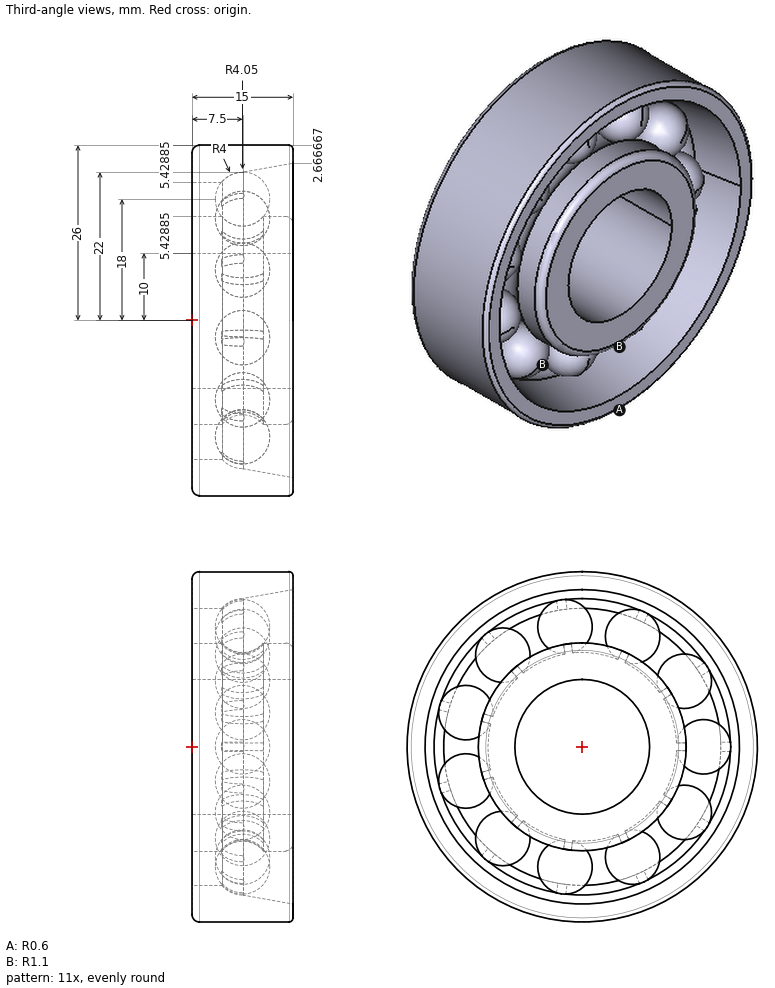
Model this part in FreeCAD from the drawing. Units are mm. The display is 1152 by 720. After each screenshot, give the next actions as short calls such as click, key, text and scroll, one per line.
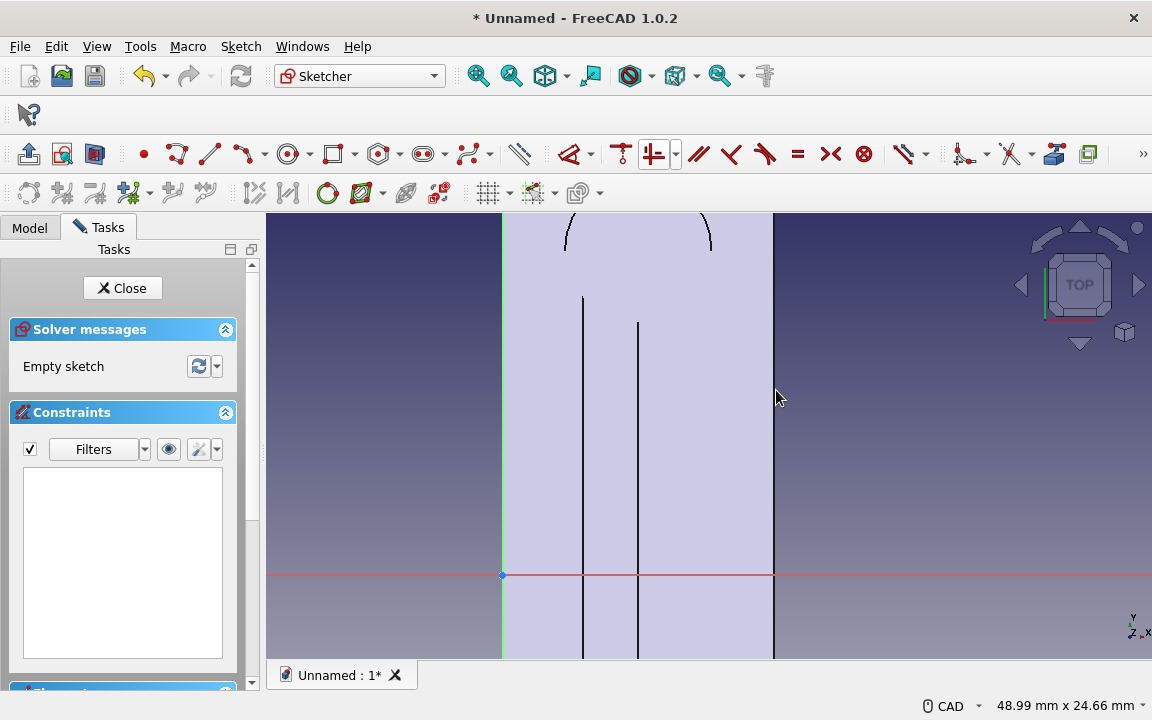
key(g)
key(m)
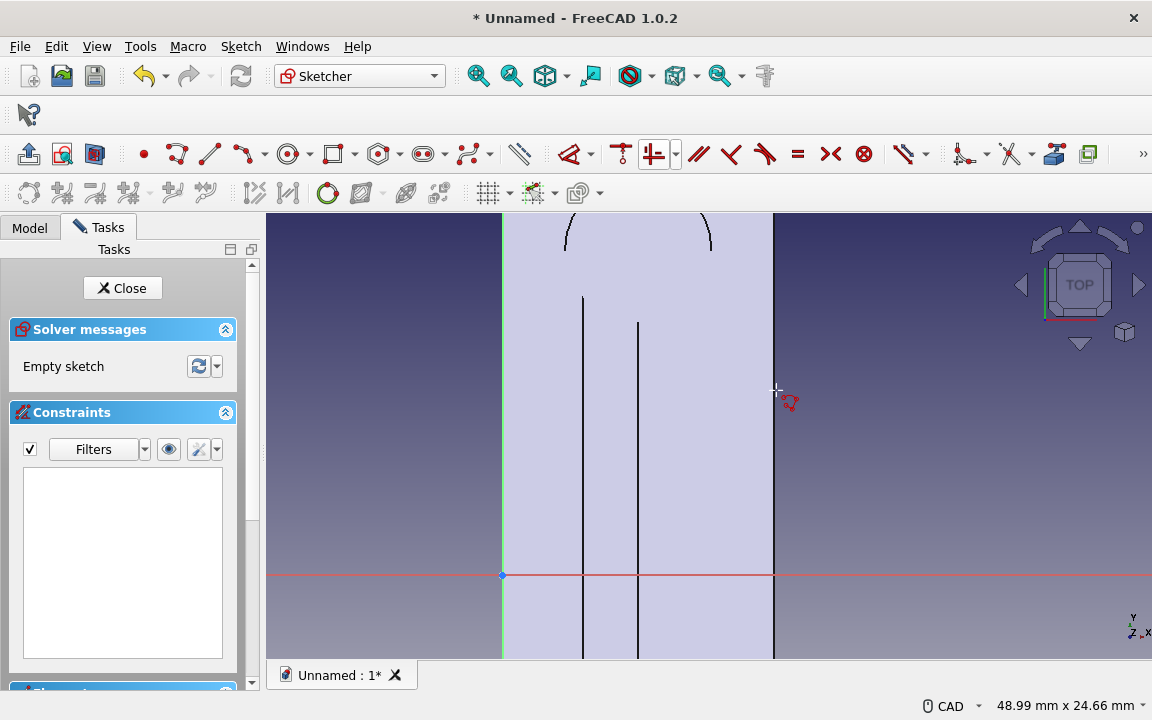
click(583, 296)
click(503, 296)
click(512, 394)
click(774, 394)
click(774, 296)
click(694, 296)
right_click(694, 296)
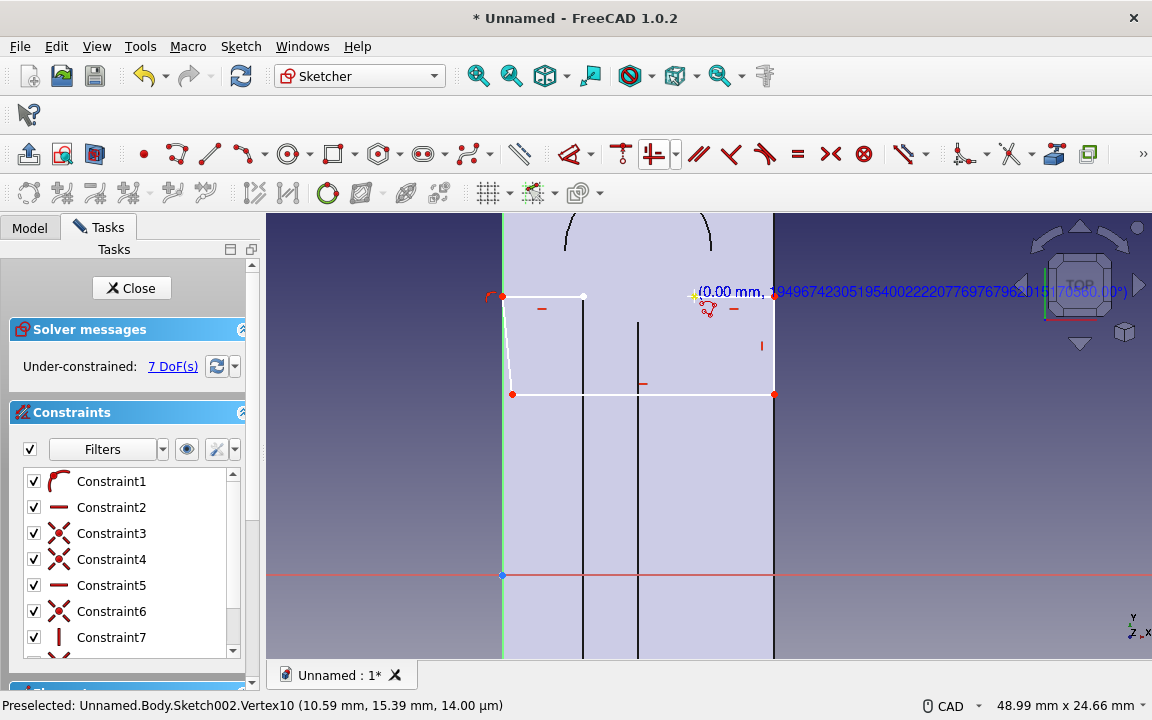
click(242, 154)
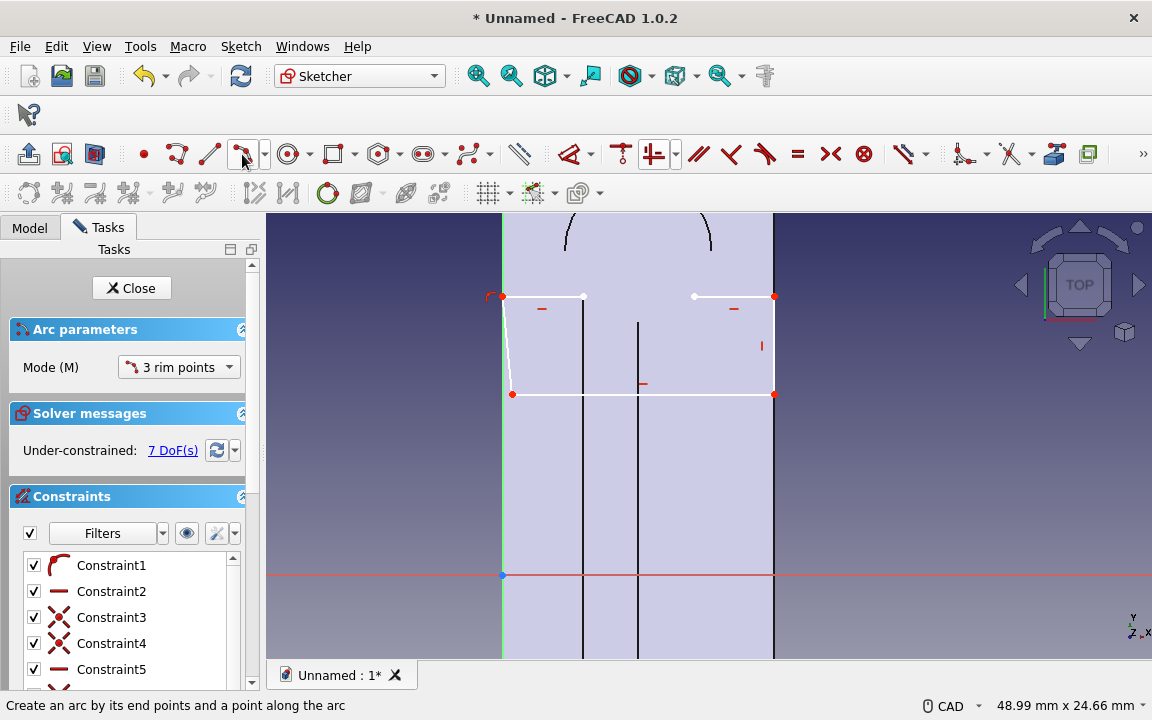
click(694, 297)
click(583, 297)
click(638, 322)
key(Escape)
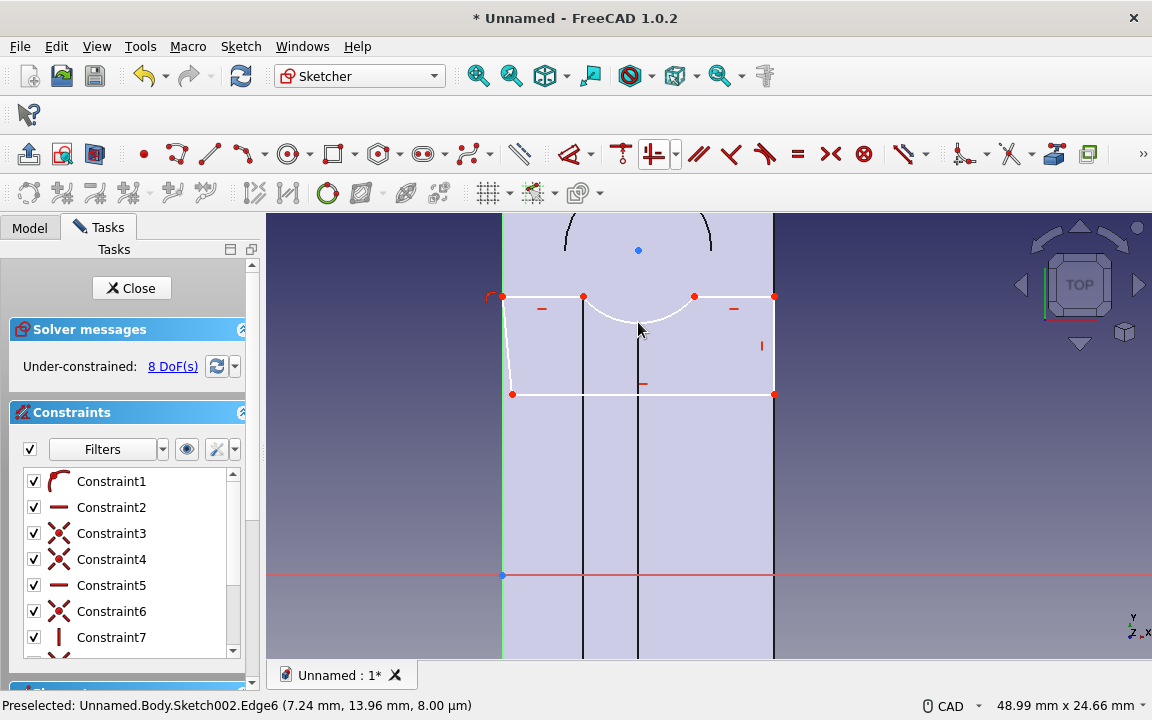
click(505, 326)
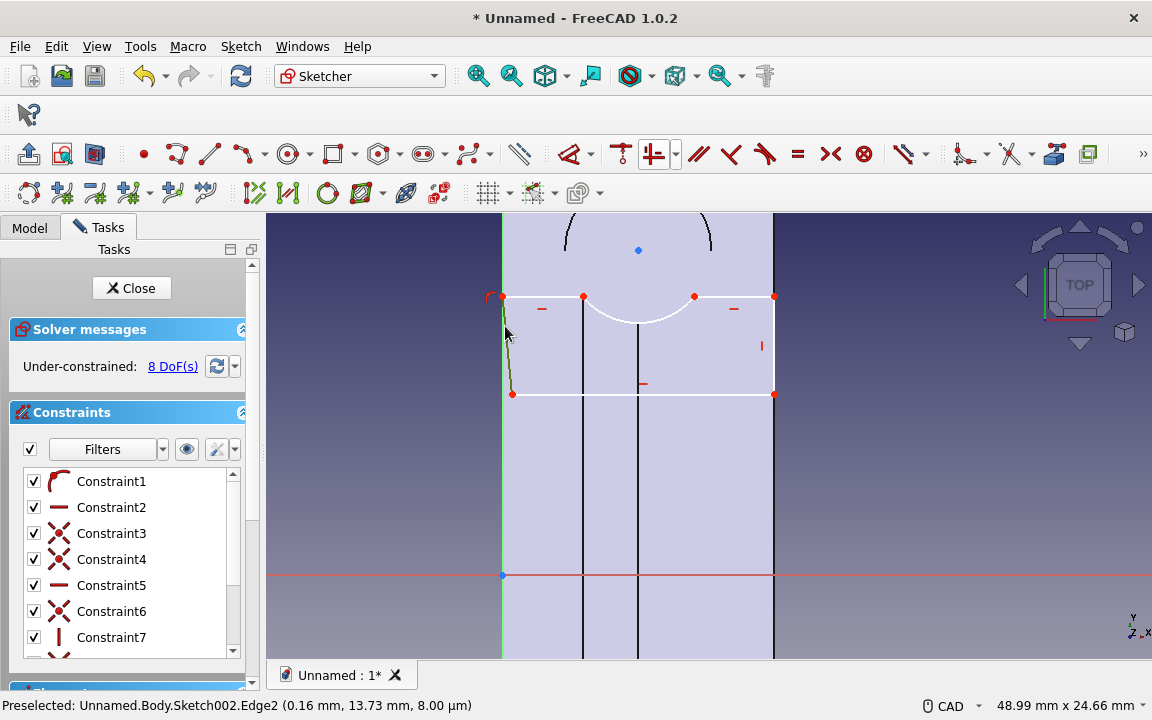
click(676, 154)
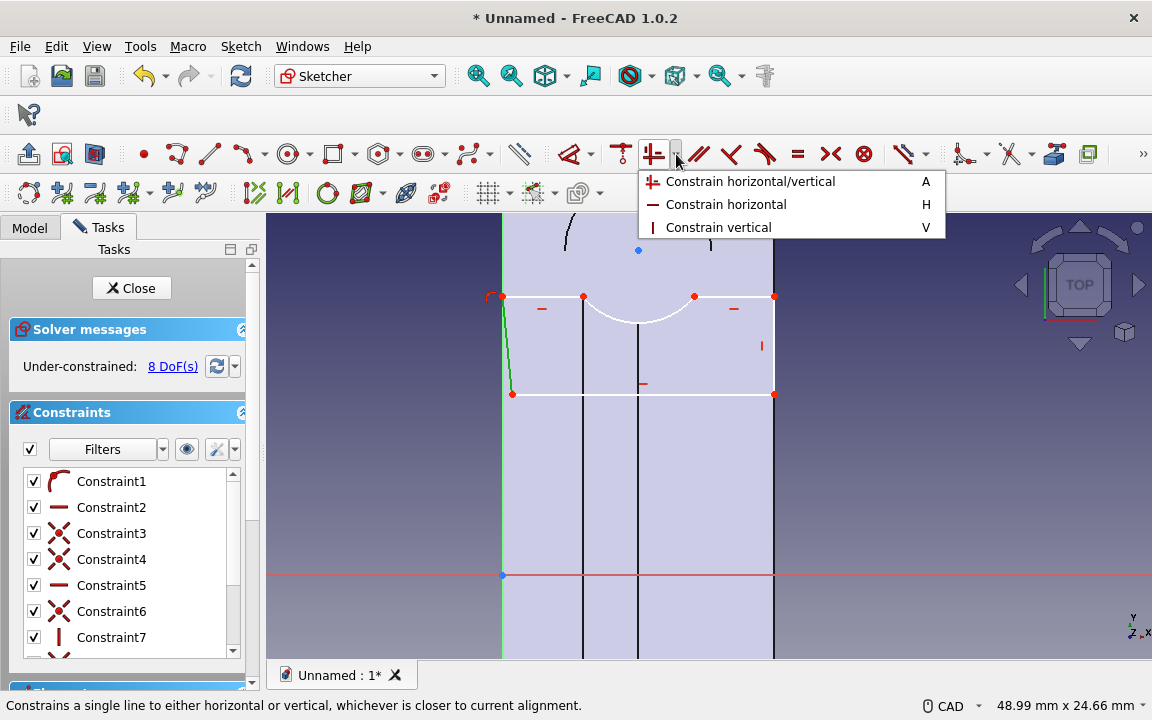
click(792, 228)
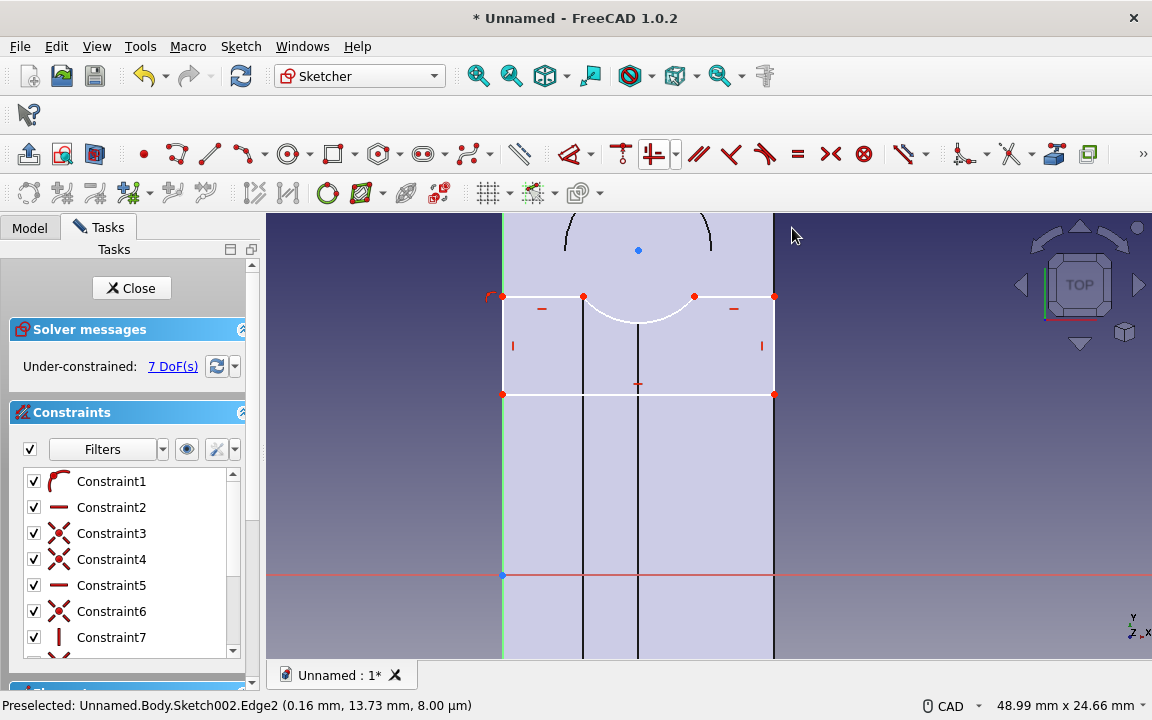
click(568, 154)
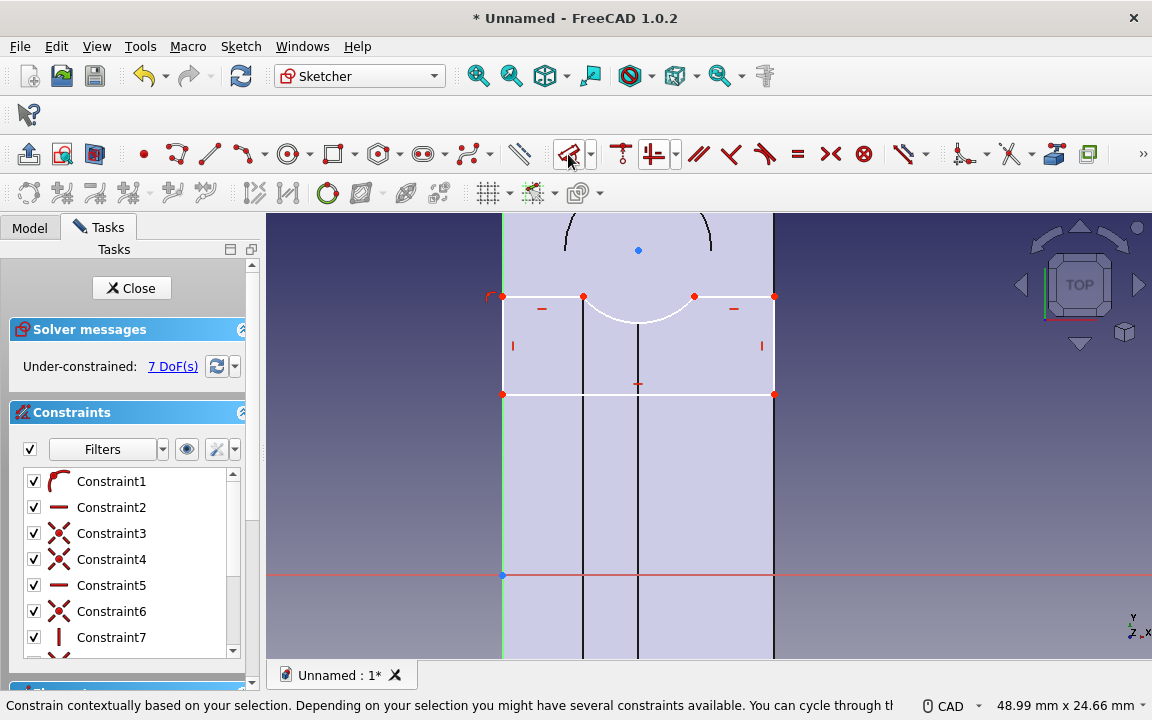
click(614, 319)
click(603, 349)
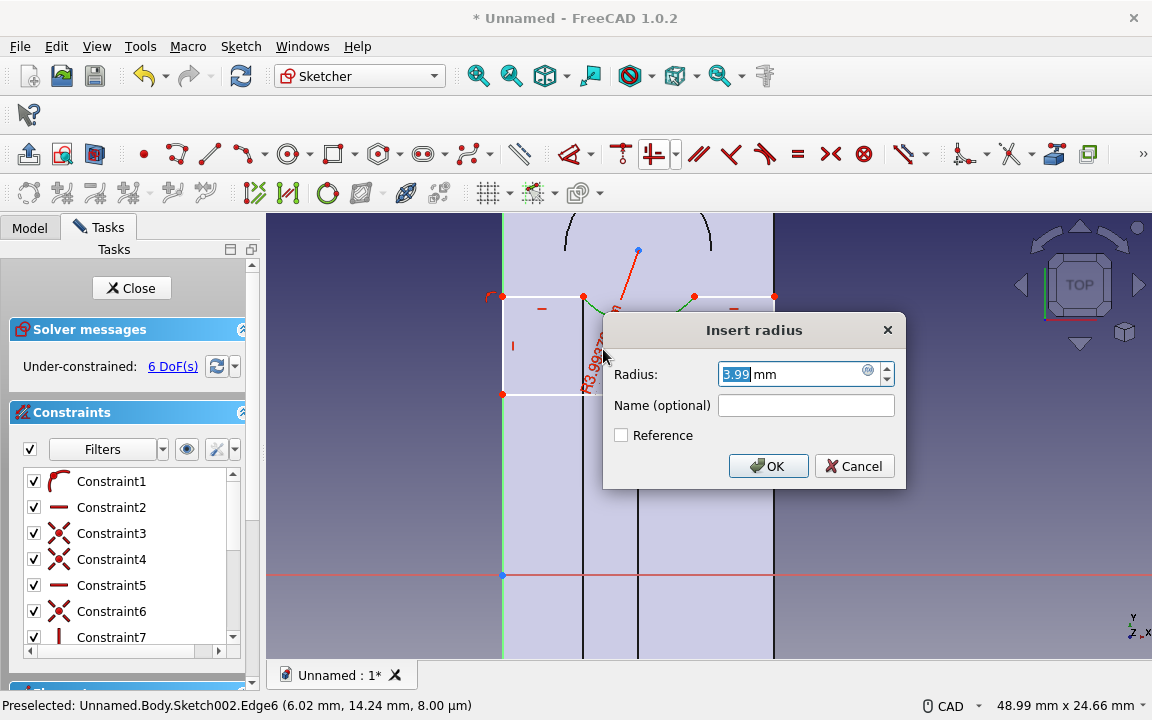
text(4)
key(Return)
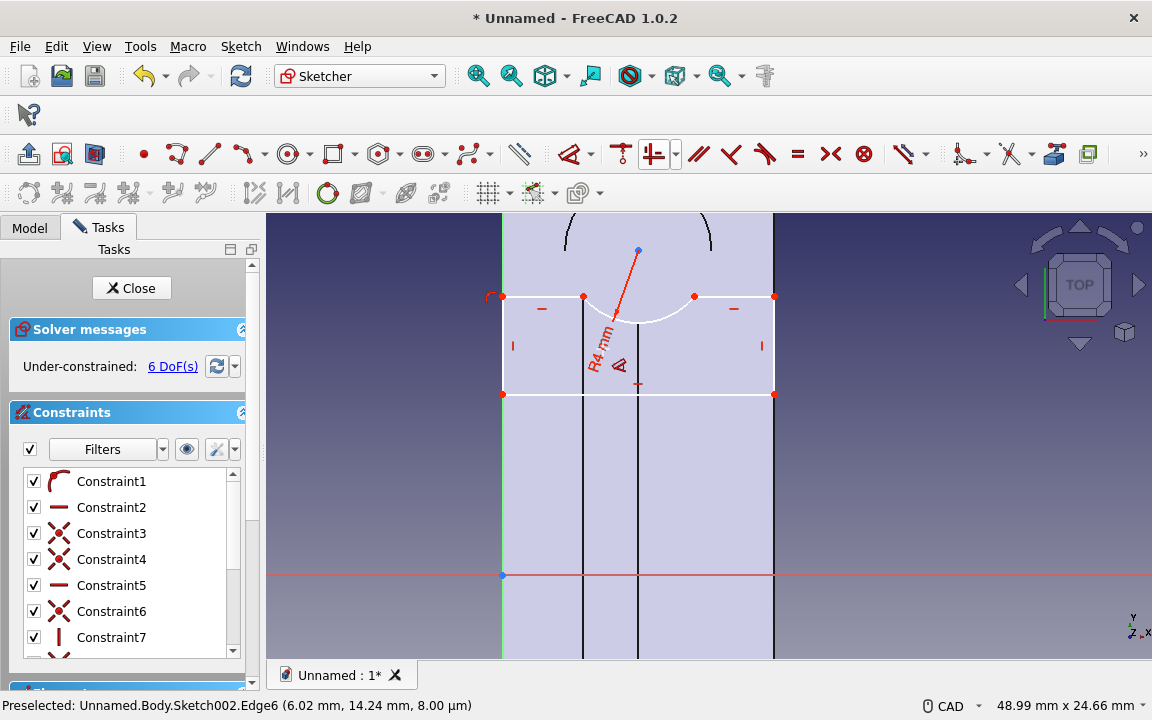
click(584, 395)
click(701, 361)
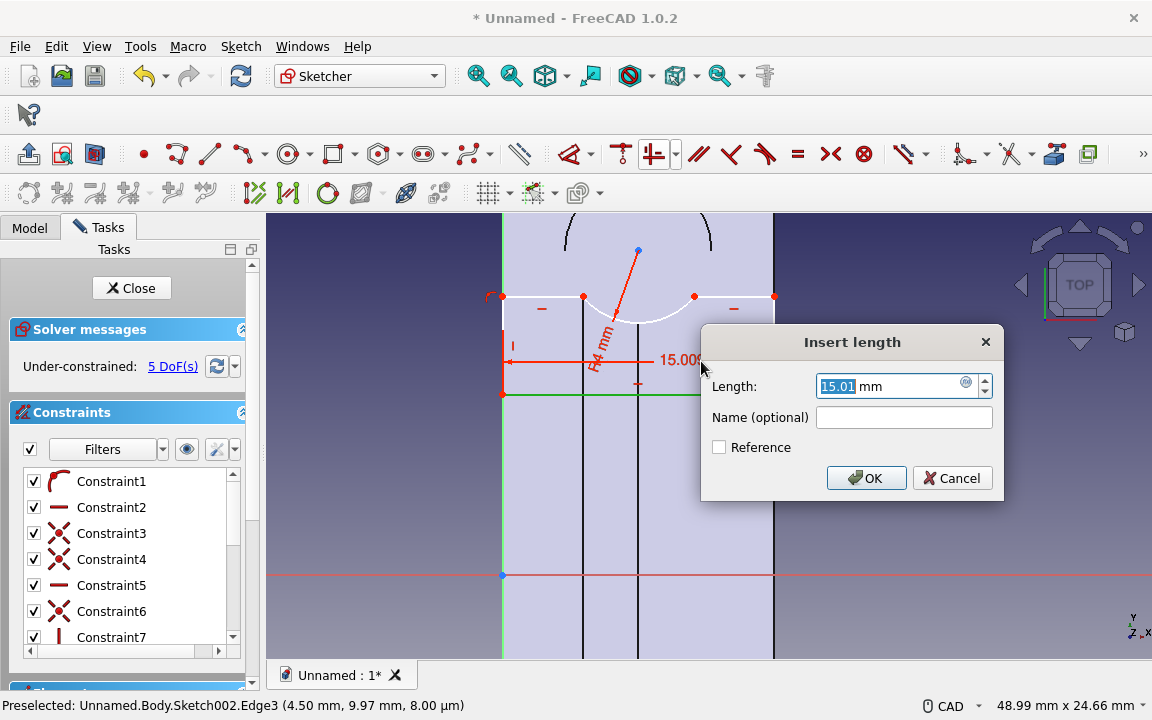
text(15)
key(Return)